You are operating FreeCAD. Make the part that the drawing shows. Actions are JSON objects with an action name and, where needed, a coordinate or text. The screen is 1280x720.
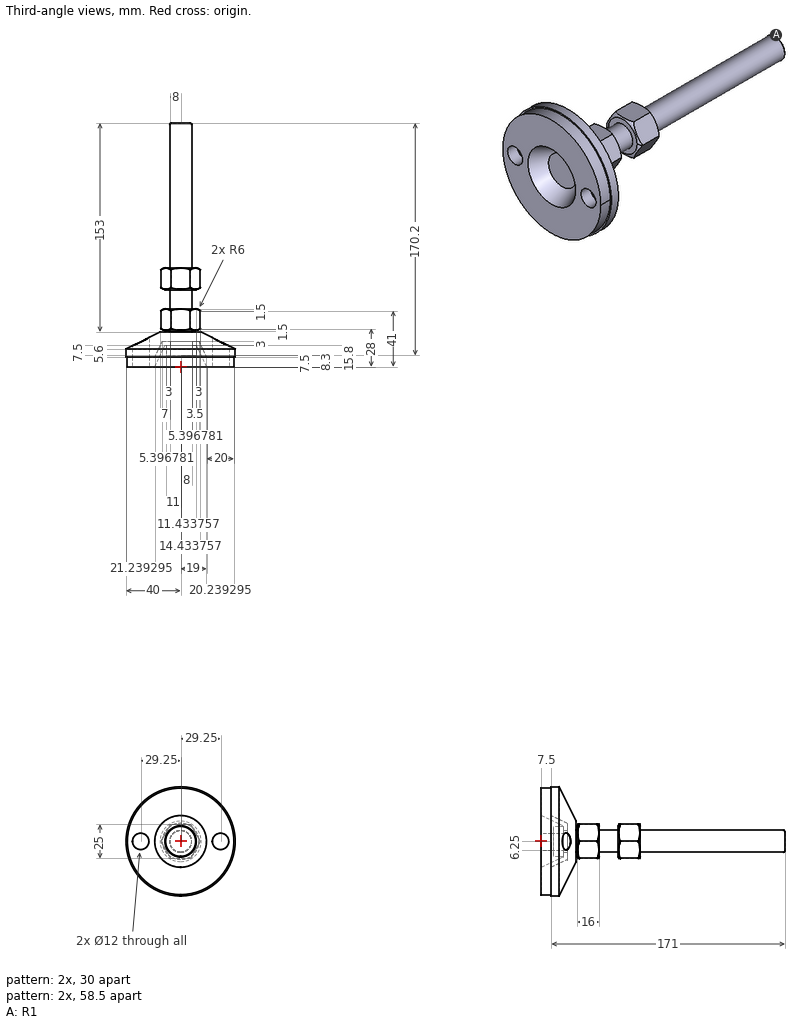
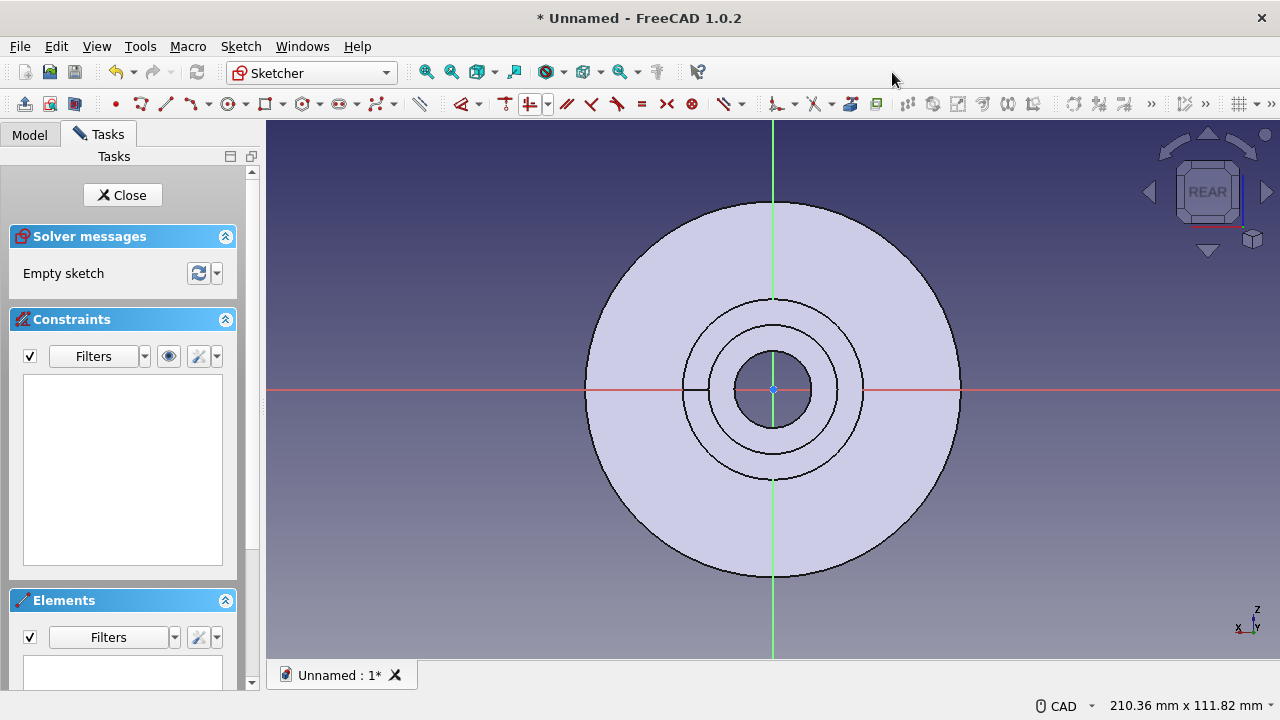
{"action": "scroll", "coordinate": [856, 389], "scroll_direction": "up", "scroll_amount": 3}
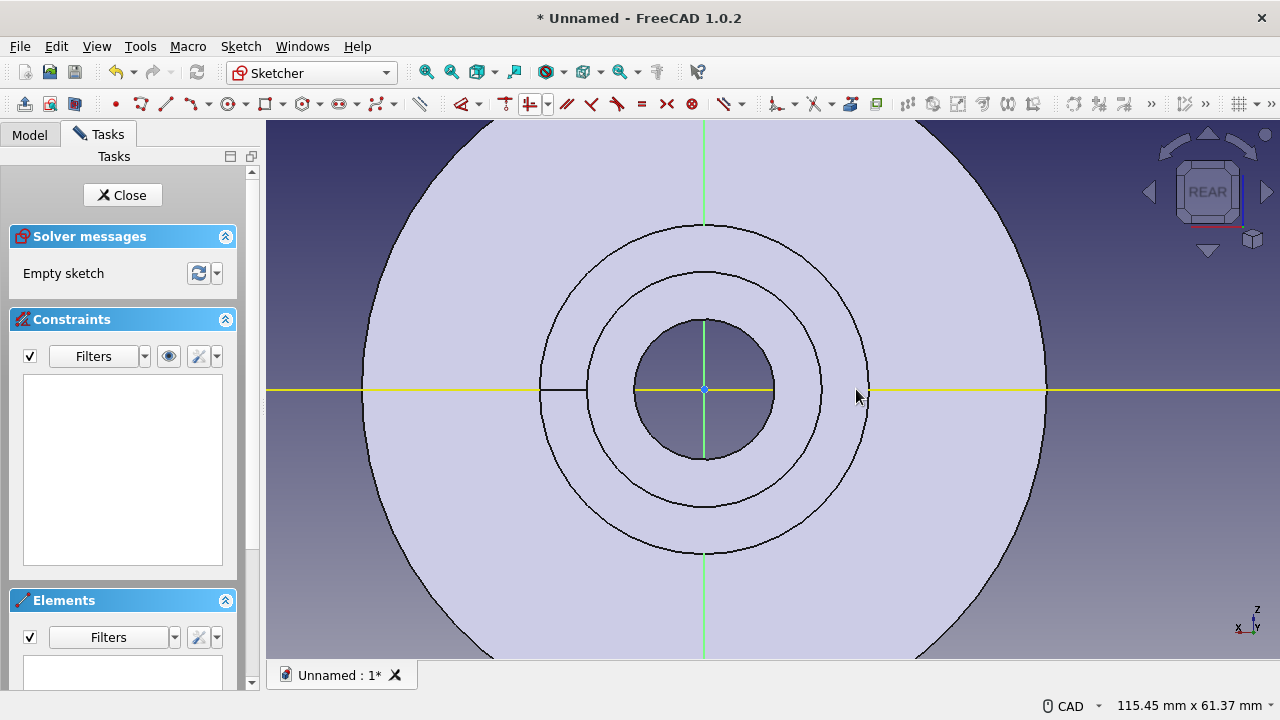
{"action": "left_click", "coordinate": [228, 104]}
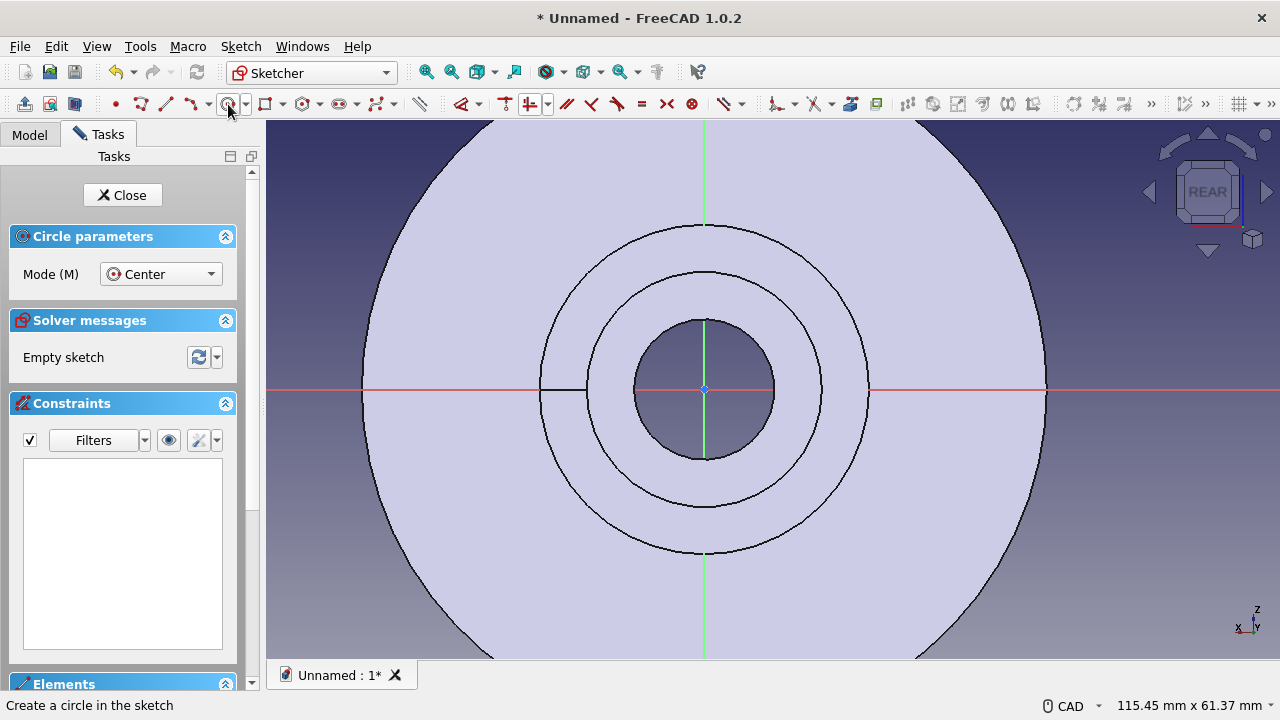
{"action": "left_click", "coordinate": [961, 389]}
{"action": "left_click", "coordinate": [998, 352]}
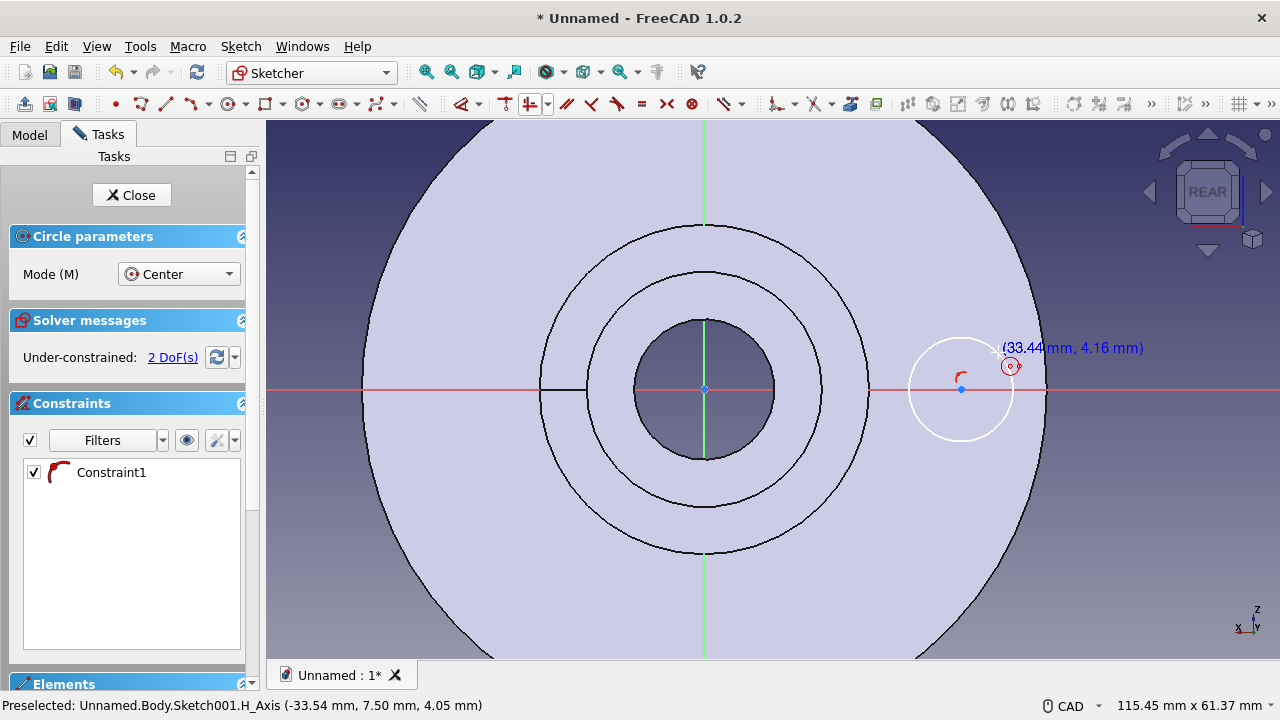
{"action": "left_click", "coordinate": [447, 389]}
{"action": "left_click", "coordinate": [485, 352]}
{"action": "key", "text": "Escape"}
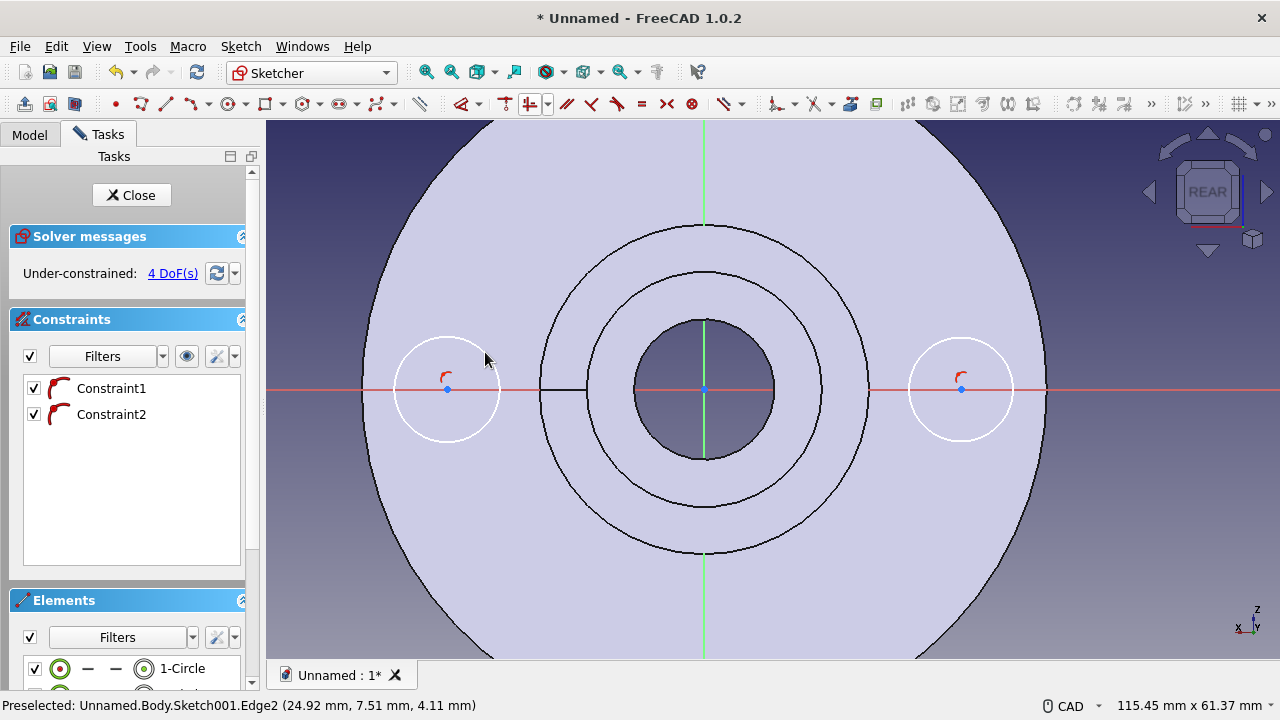
{"action": "left_click", "coordinate": [998, 353]}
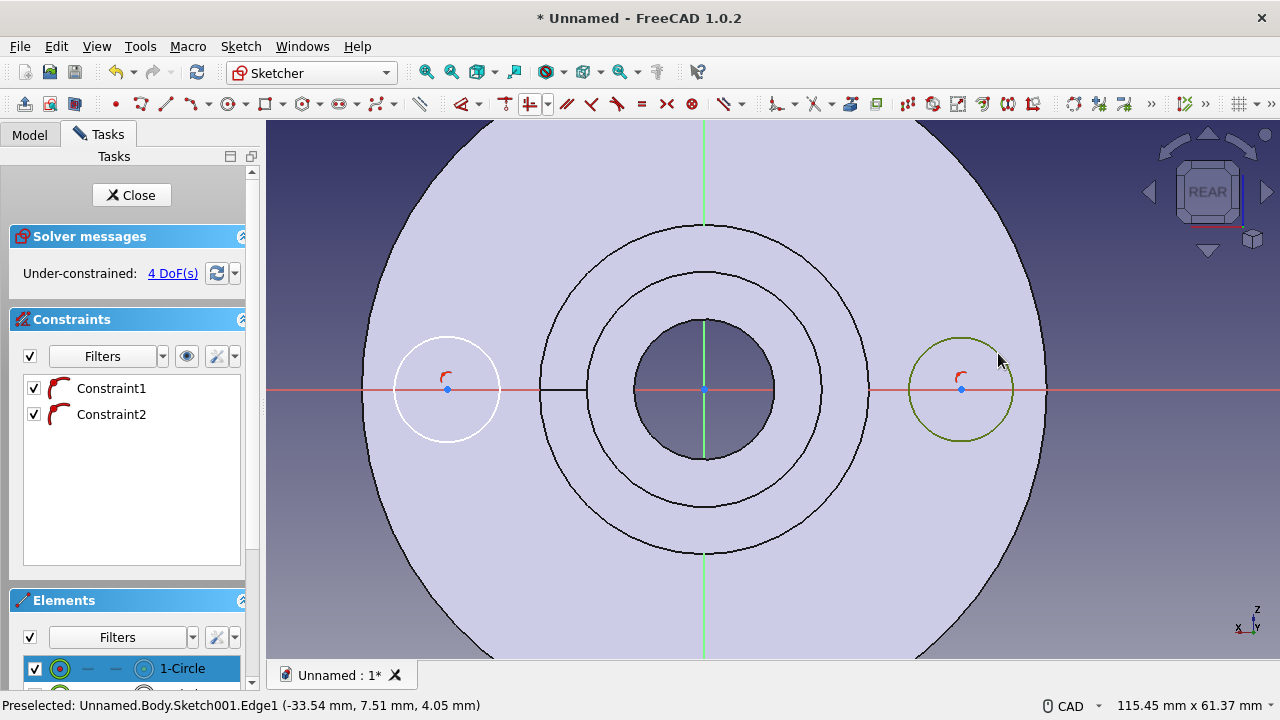
{"action": "left_click", "coordinate": [484, 352]}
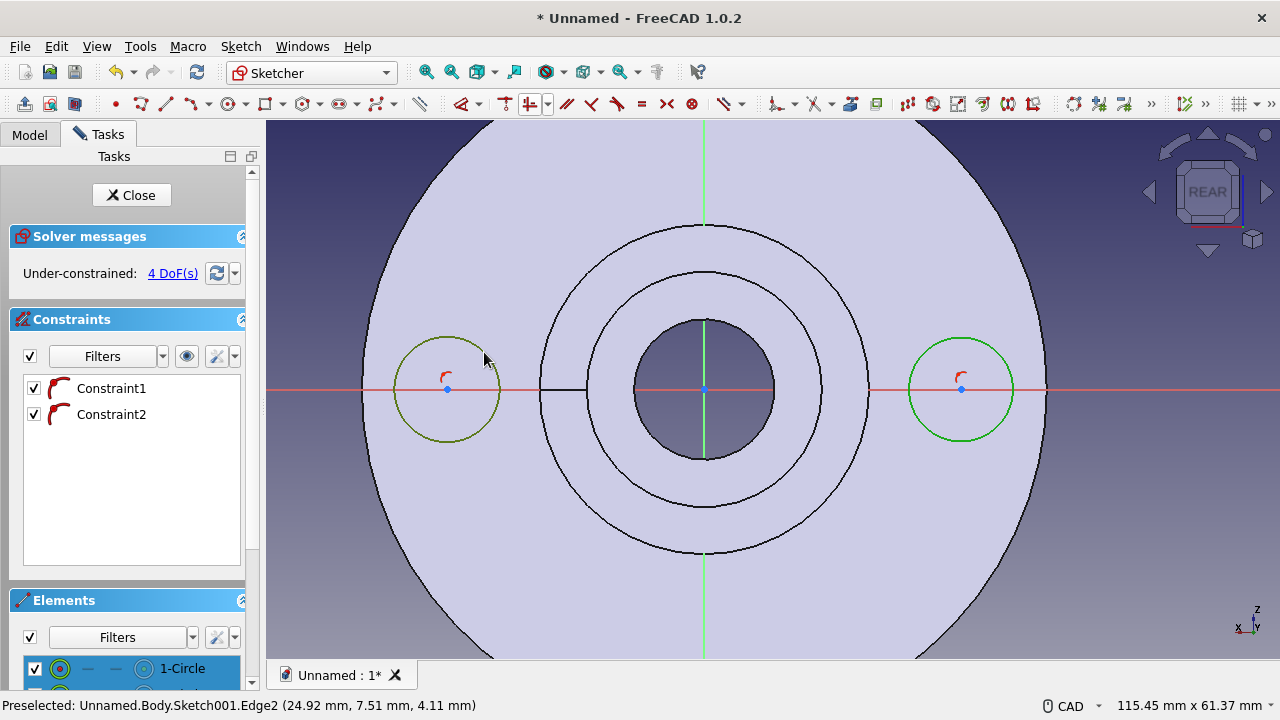
{"action": "left_click", "coordinate": [642, 104]}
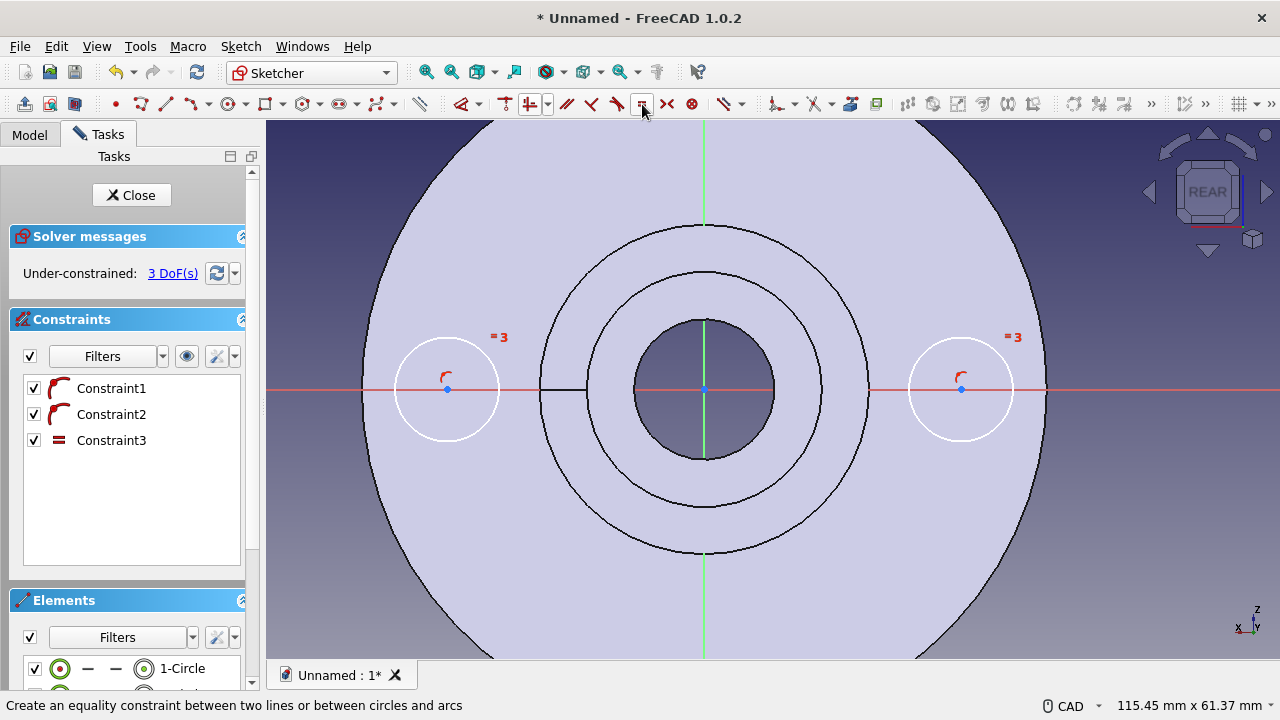
{"action": "left_click", "coordinate": [460, 104]}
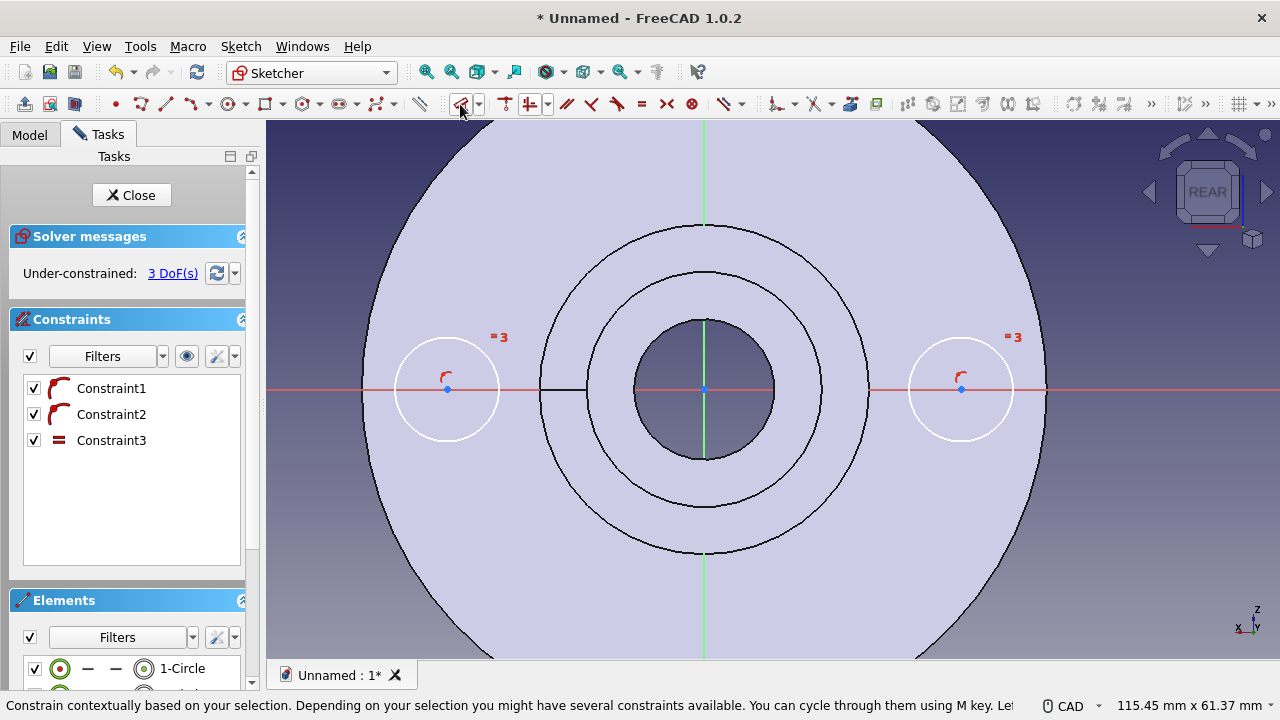
{"action": "left_click", "coordinate": [998, 353]}
{"action": "left_click", "coordinate": [1021, 331]}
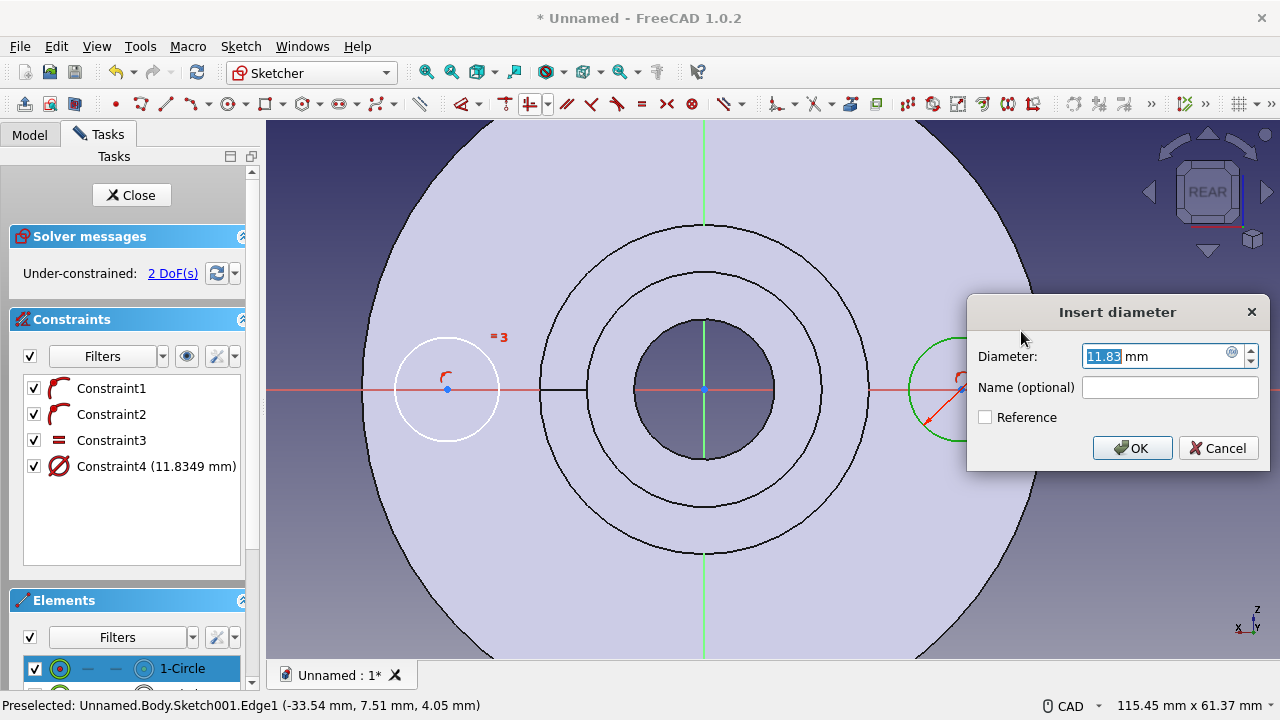
{"action": "type", "text": "12"}
{"action": "key", "text": "Return"}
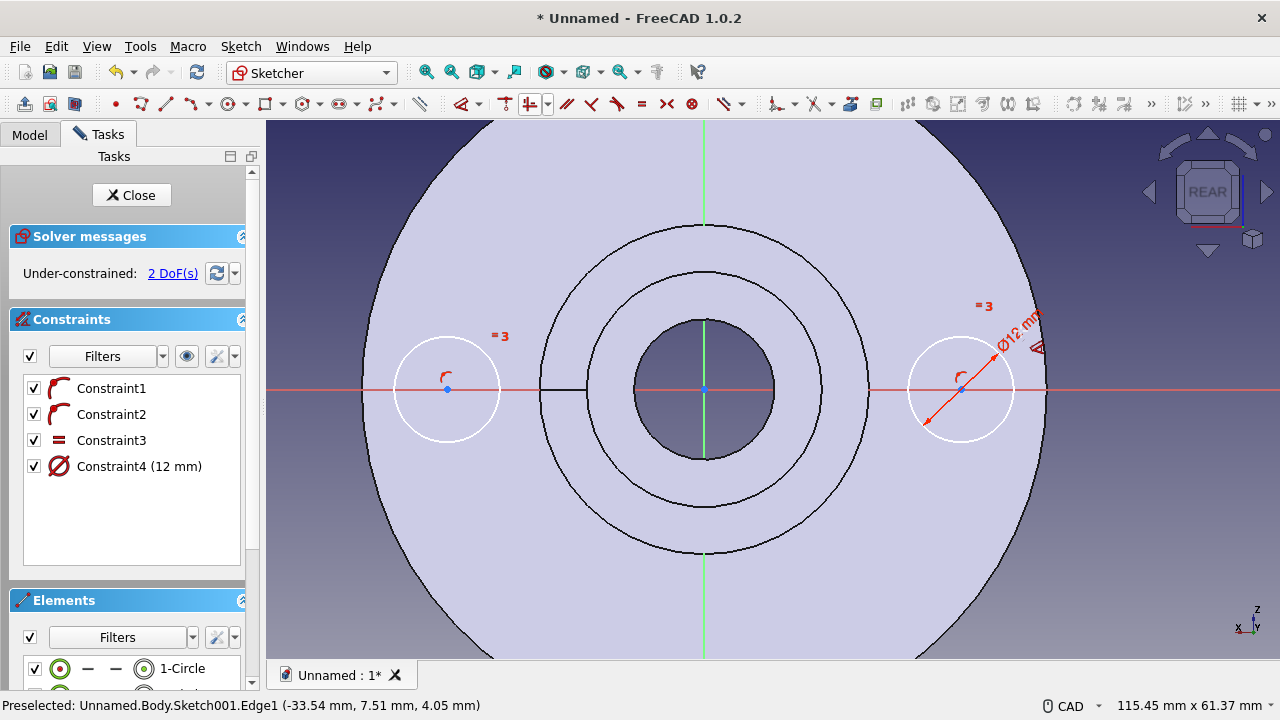
{"action": "left_click", "coordinate": [961, 389]}
{"action": "left_click", "coordinate": [833, 423]}